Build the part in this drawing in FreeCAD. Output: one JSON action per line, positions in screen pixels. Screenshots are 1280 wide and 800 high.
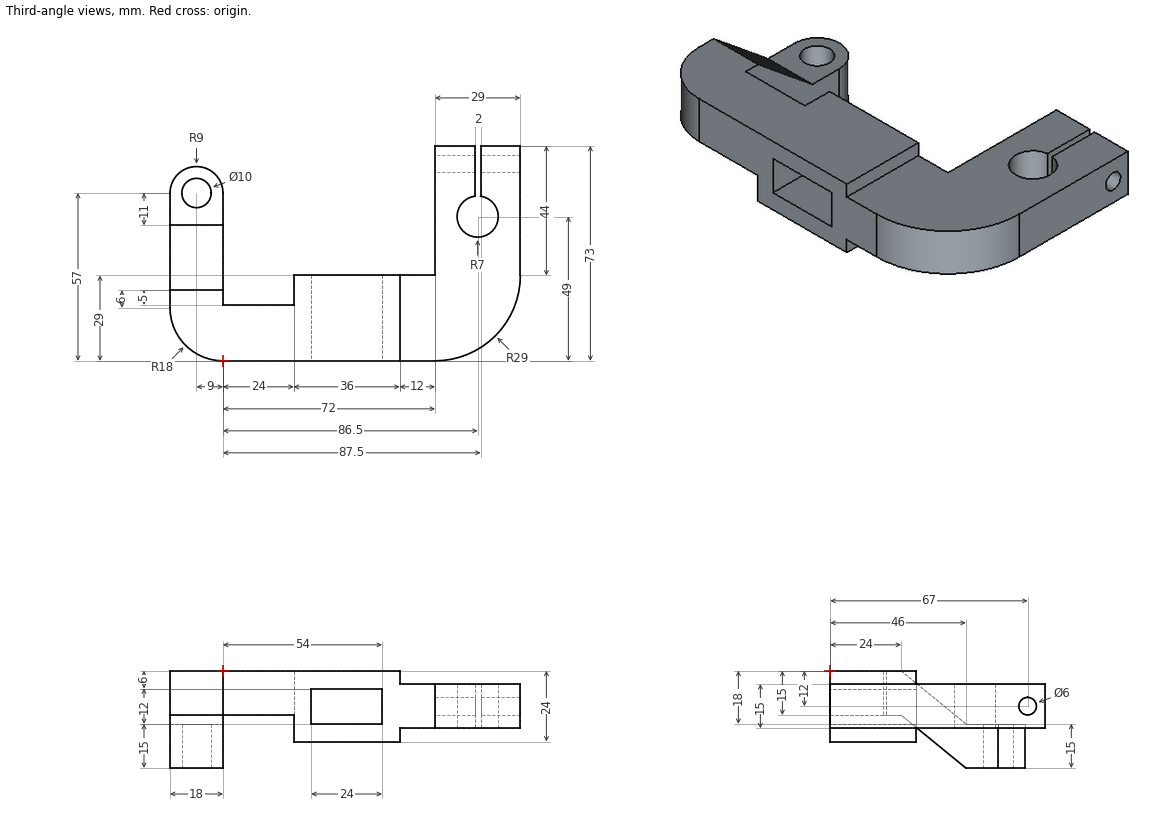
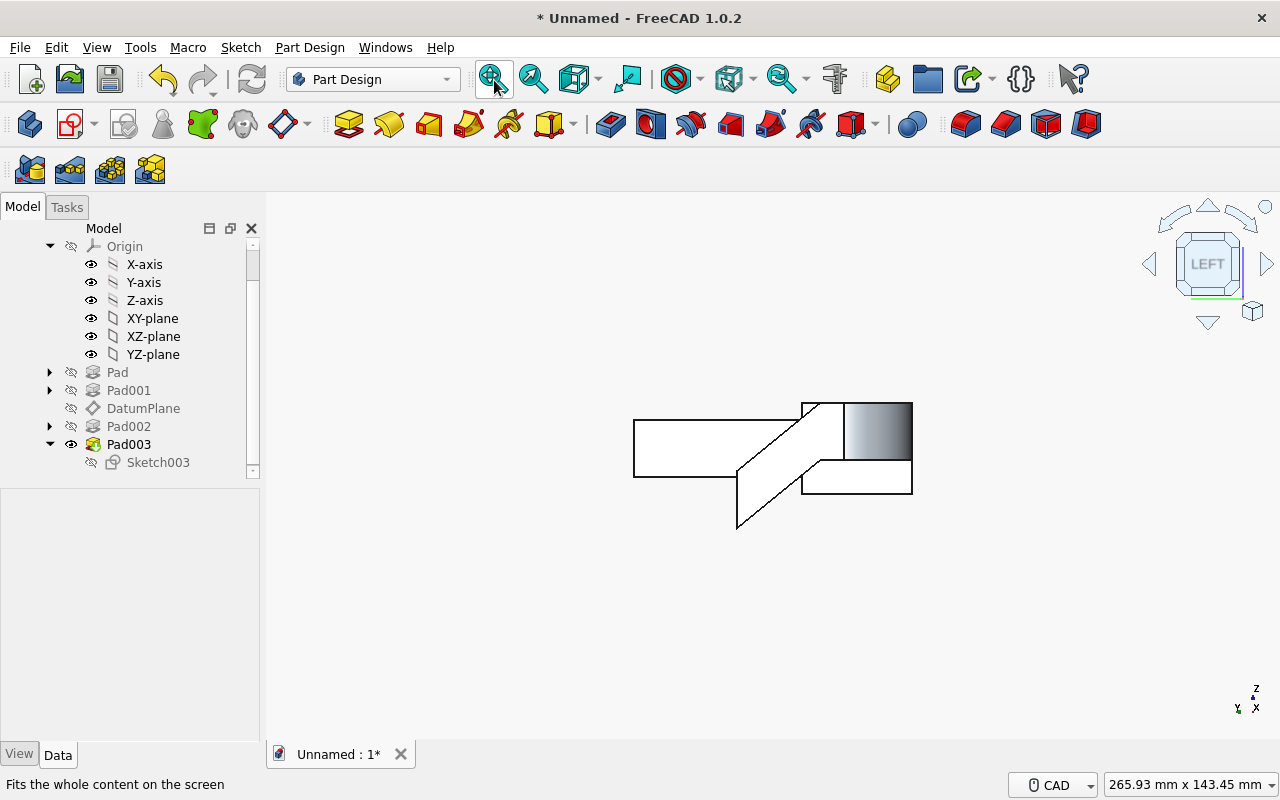
{"action": "left_click", "coordinate": [136, 318]}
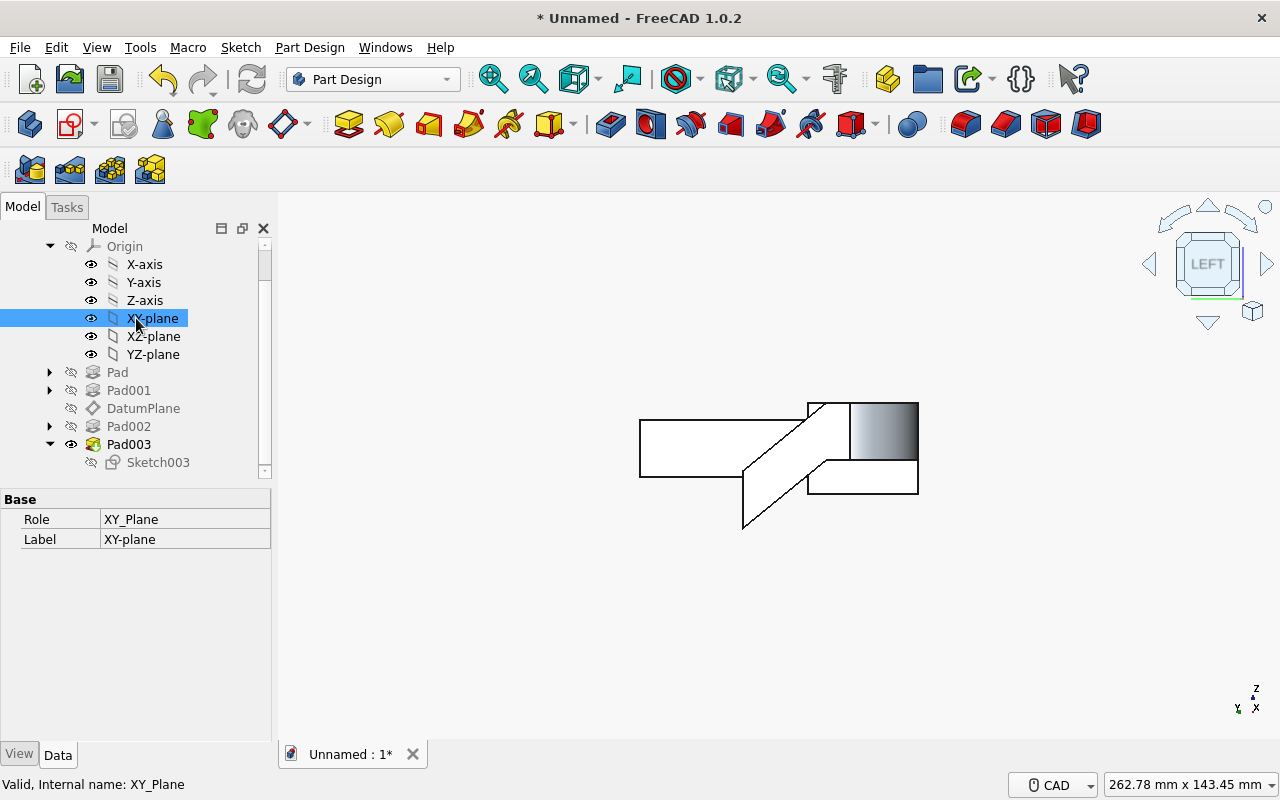
{"action": "left_click", "coordinate": [284, 124]}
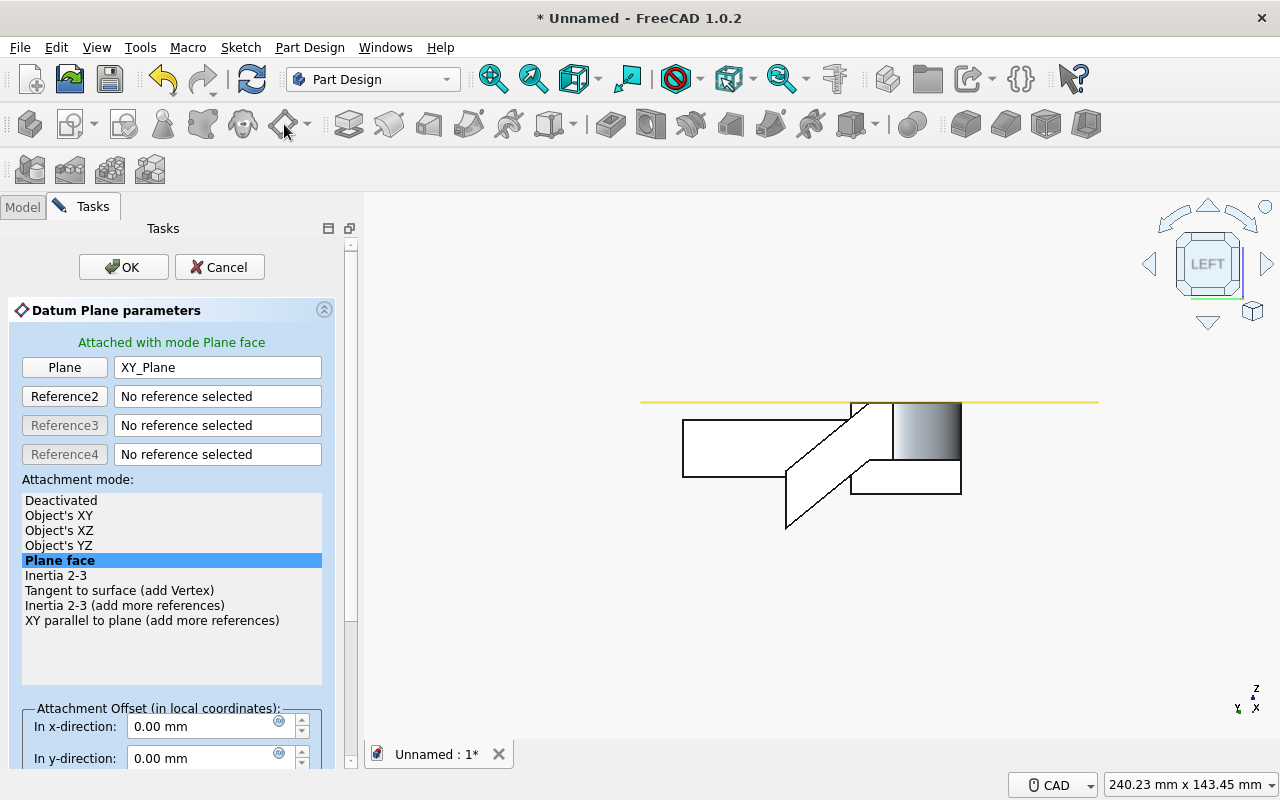
{"action": "scroll", "coordinate": [351, 503], "scroll_direction": "down", "scroll_amount": 2}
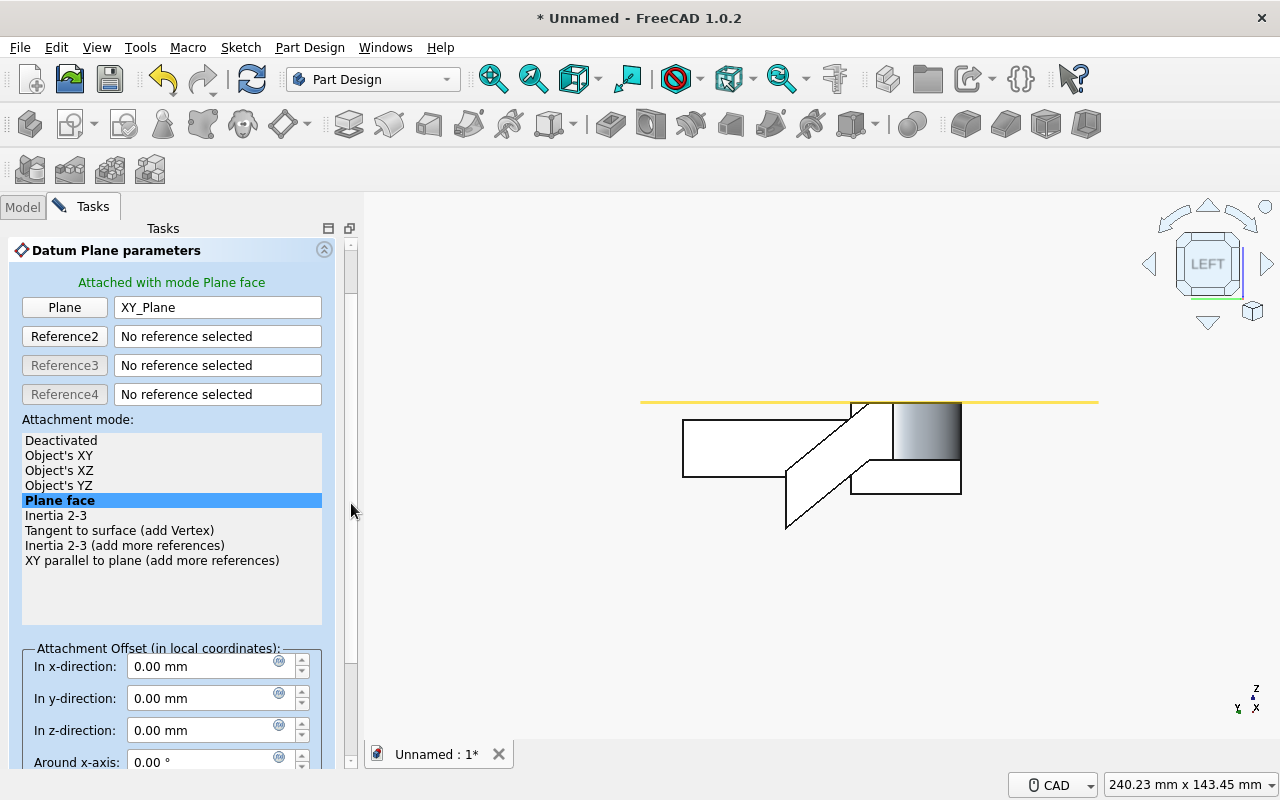
{"action": "triple_click", "coordinate": [210, 670]}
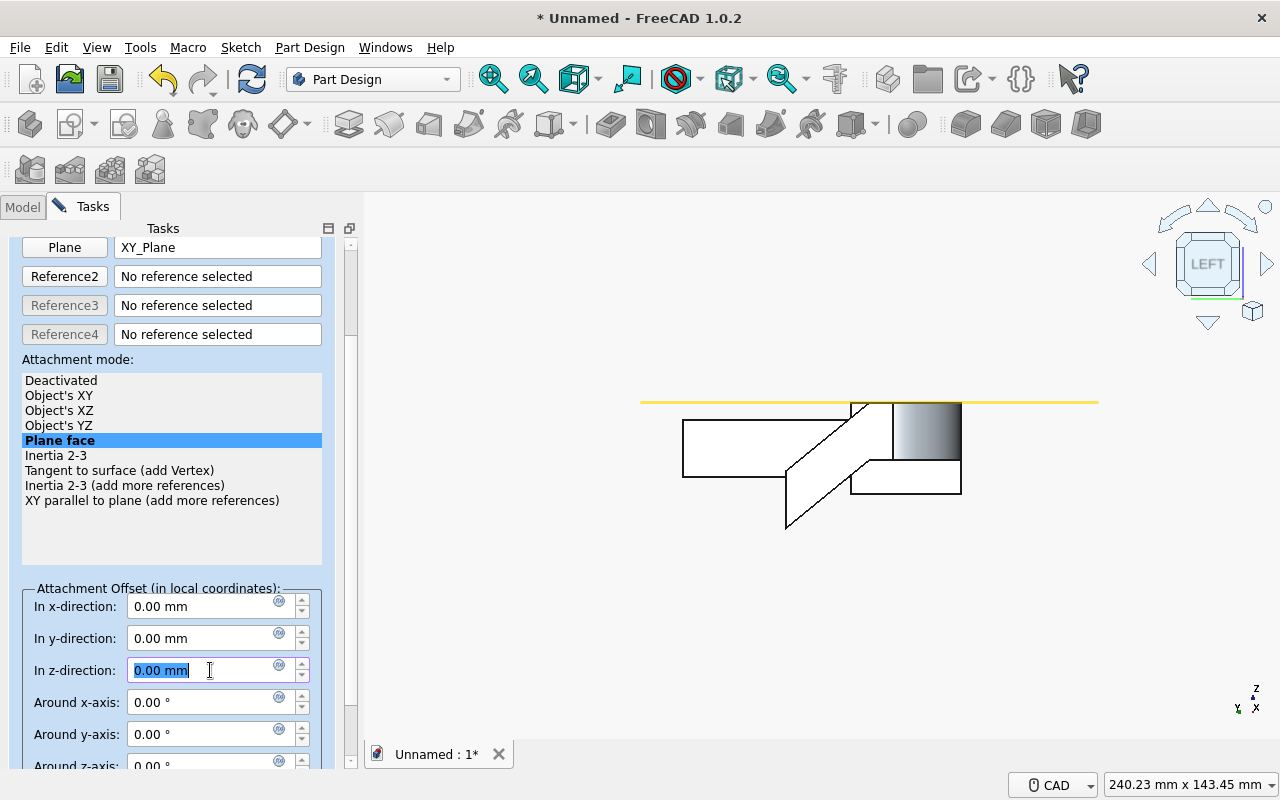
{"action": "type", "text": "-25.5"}
{"action": "key", "text": "Tab"}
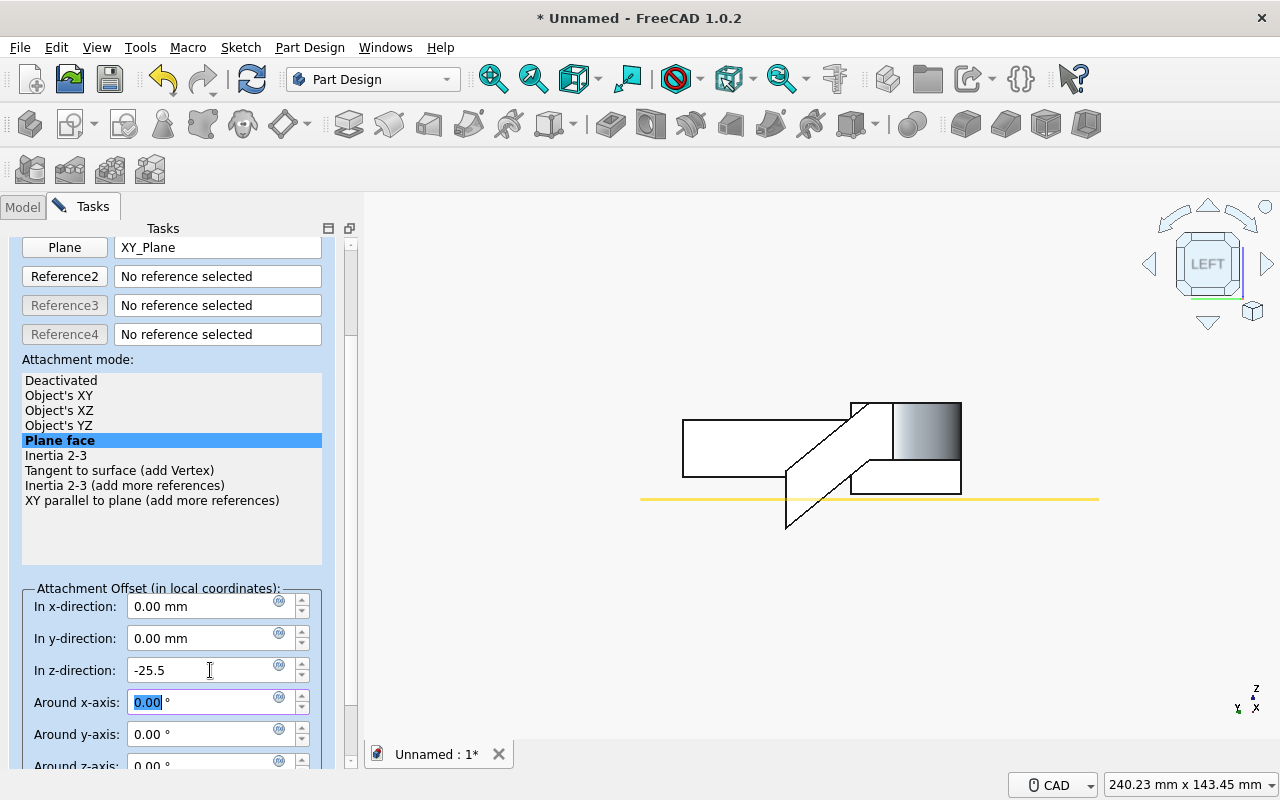
{"action": "scroll", "coordinate": [351, 503], "scroll_direction": "up", "scroll_amount": 3}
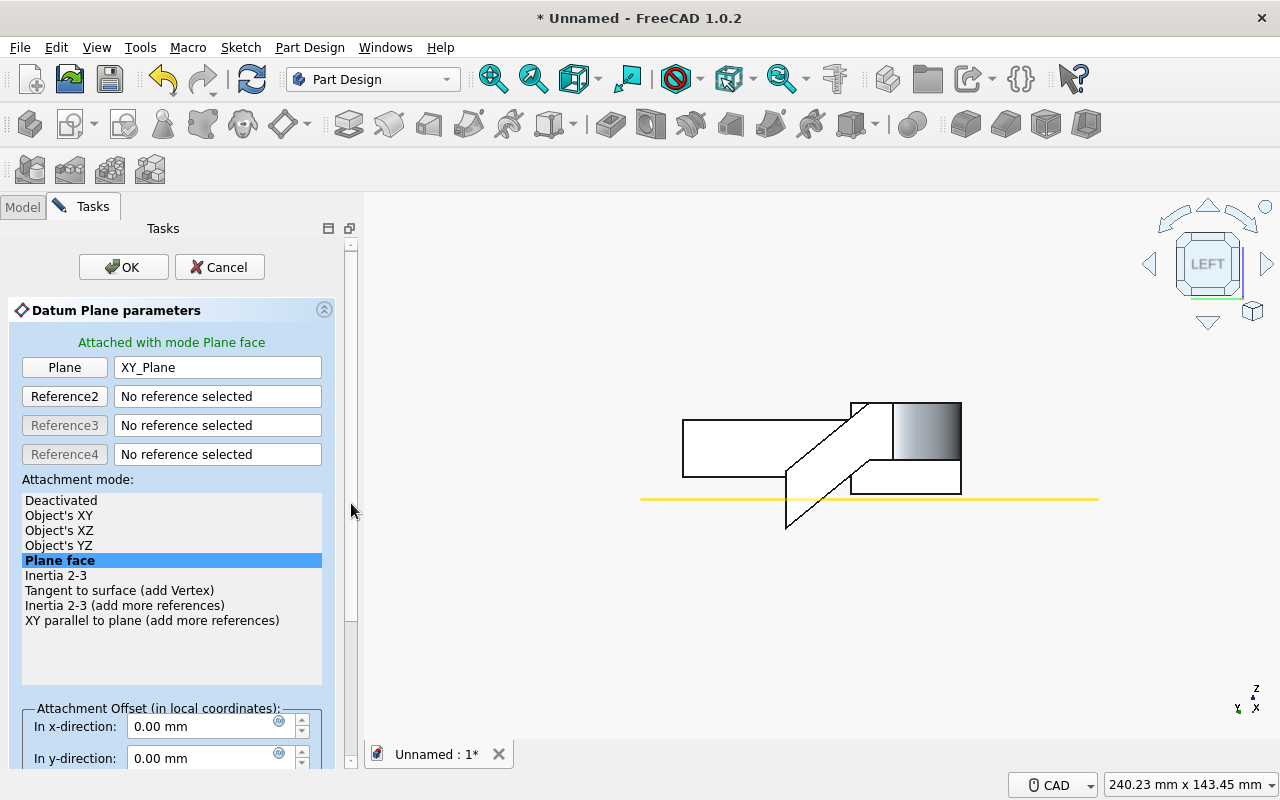
{"action": "left_click", "coordinate": [124, 267]}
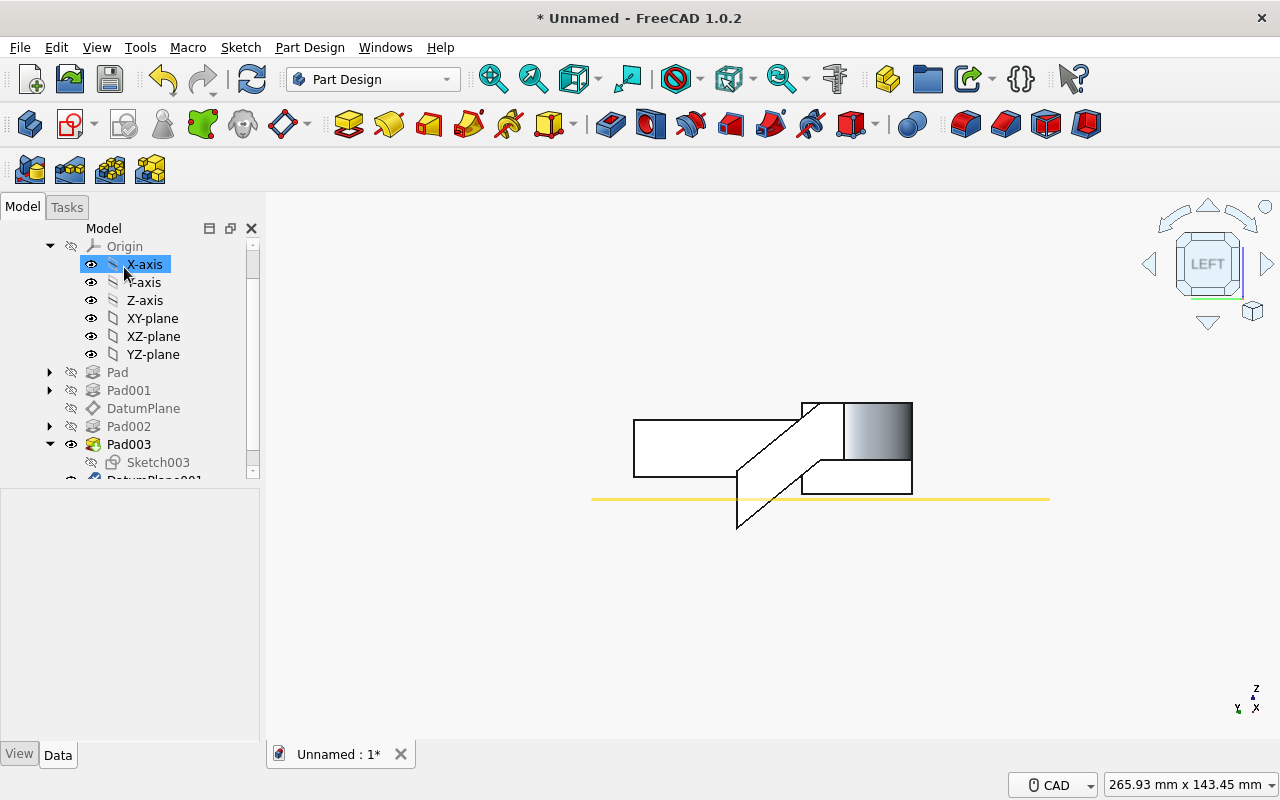
{"action": "scroll", "coordinate": [140, 350], "scroll_direction": "down", "scroll_amount": 3}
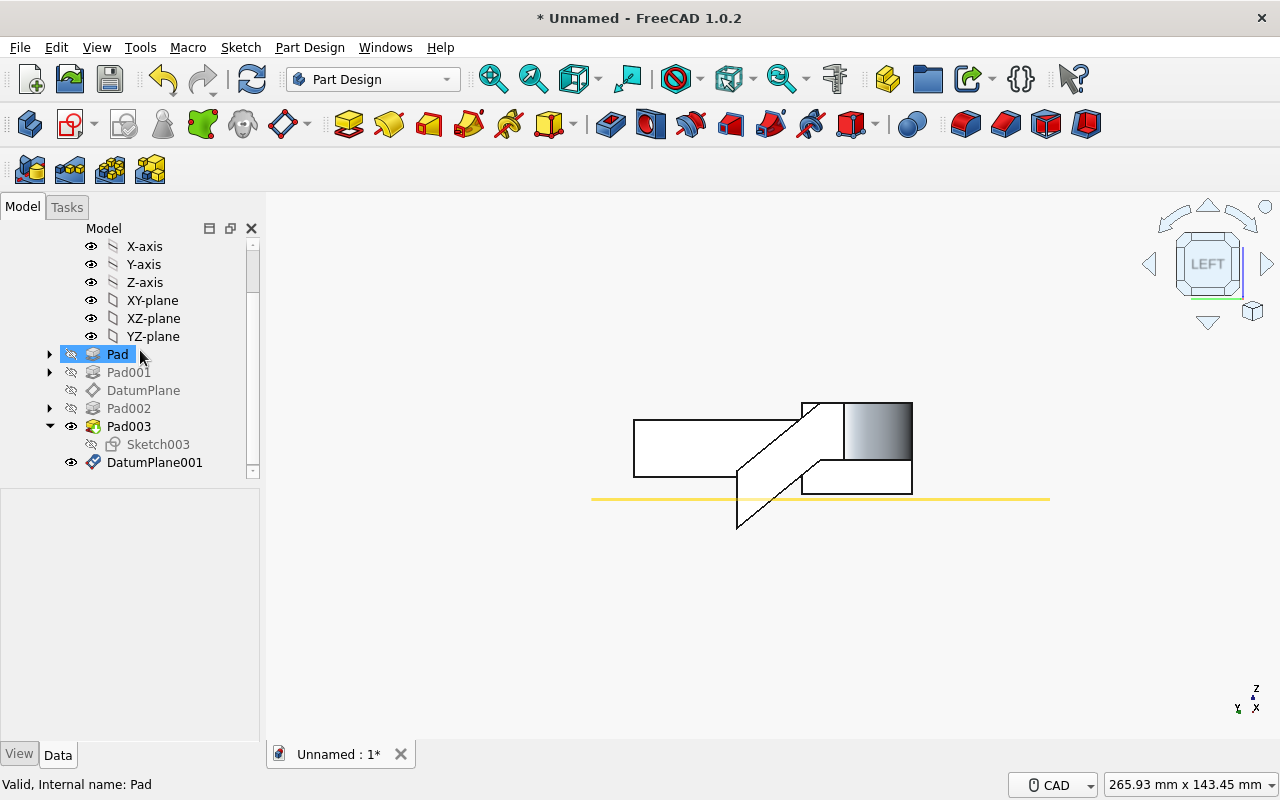
{"action": "left_click", "coordinate": [116, 462]}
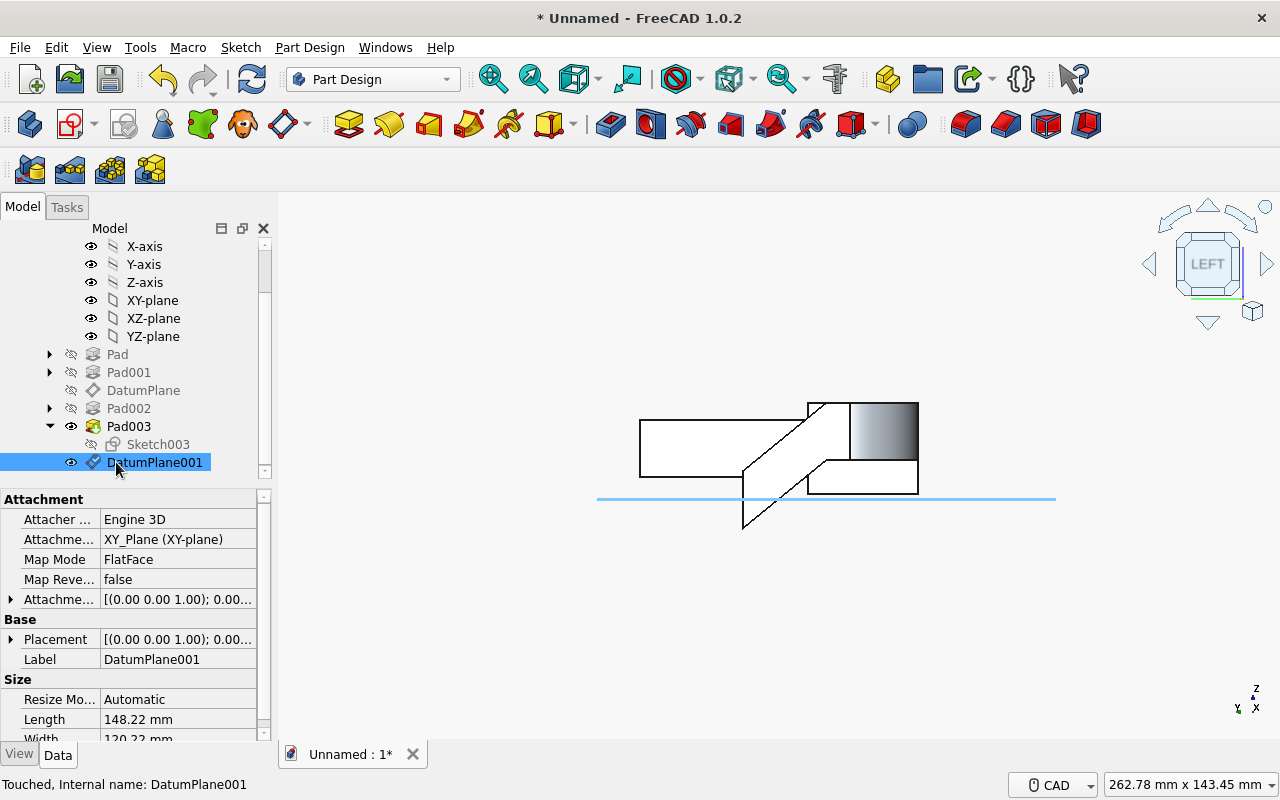
{"action": "left_click", "coordinate": [70, 124]}